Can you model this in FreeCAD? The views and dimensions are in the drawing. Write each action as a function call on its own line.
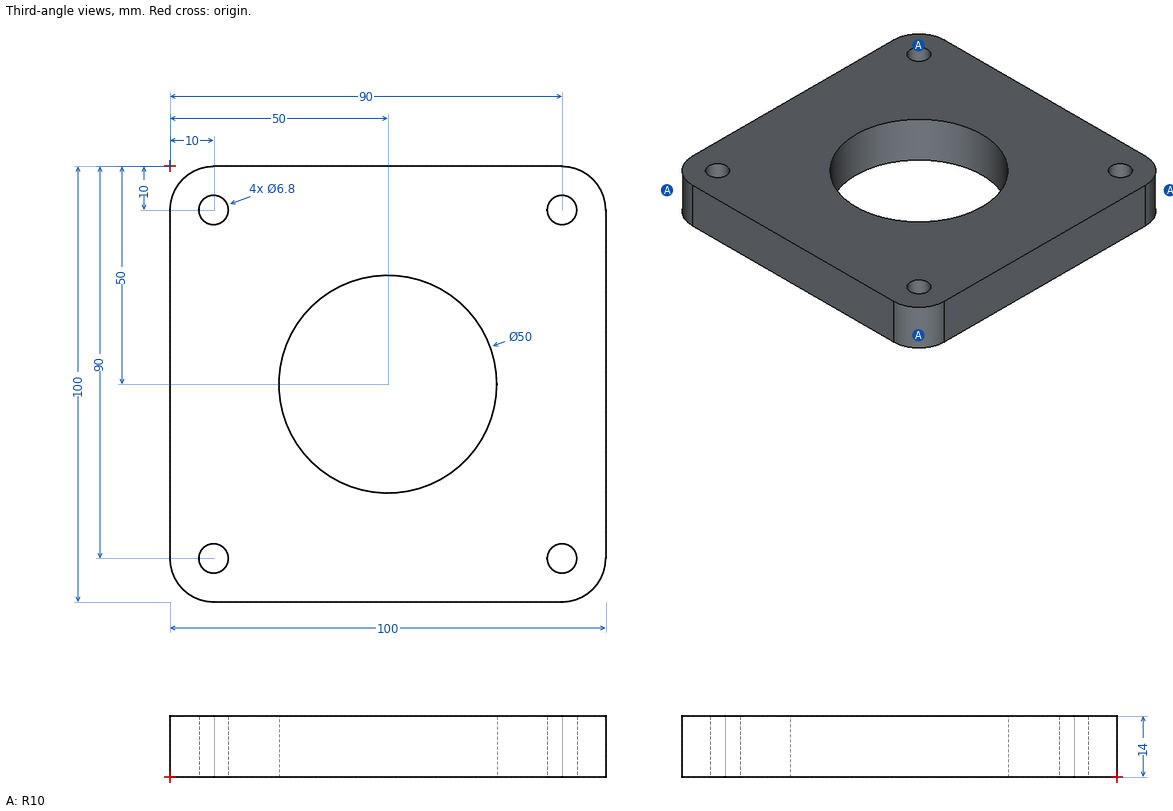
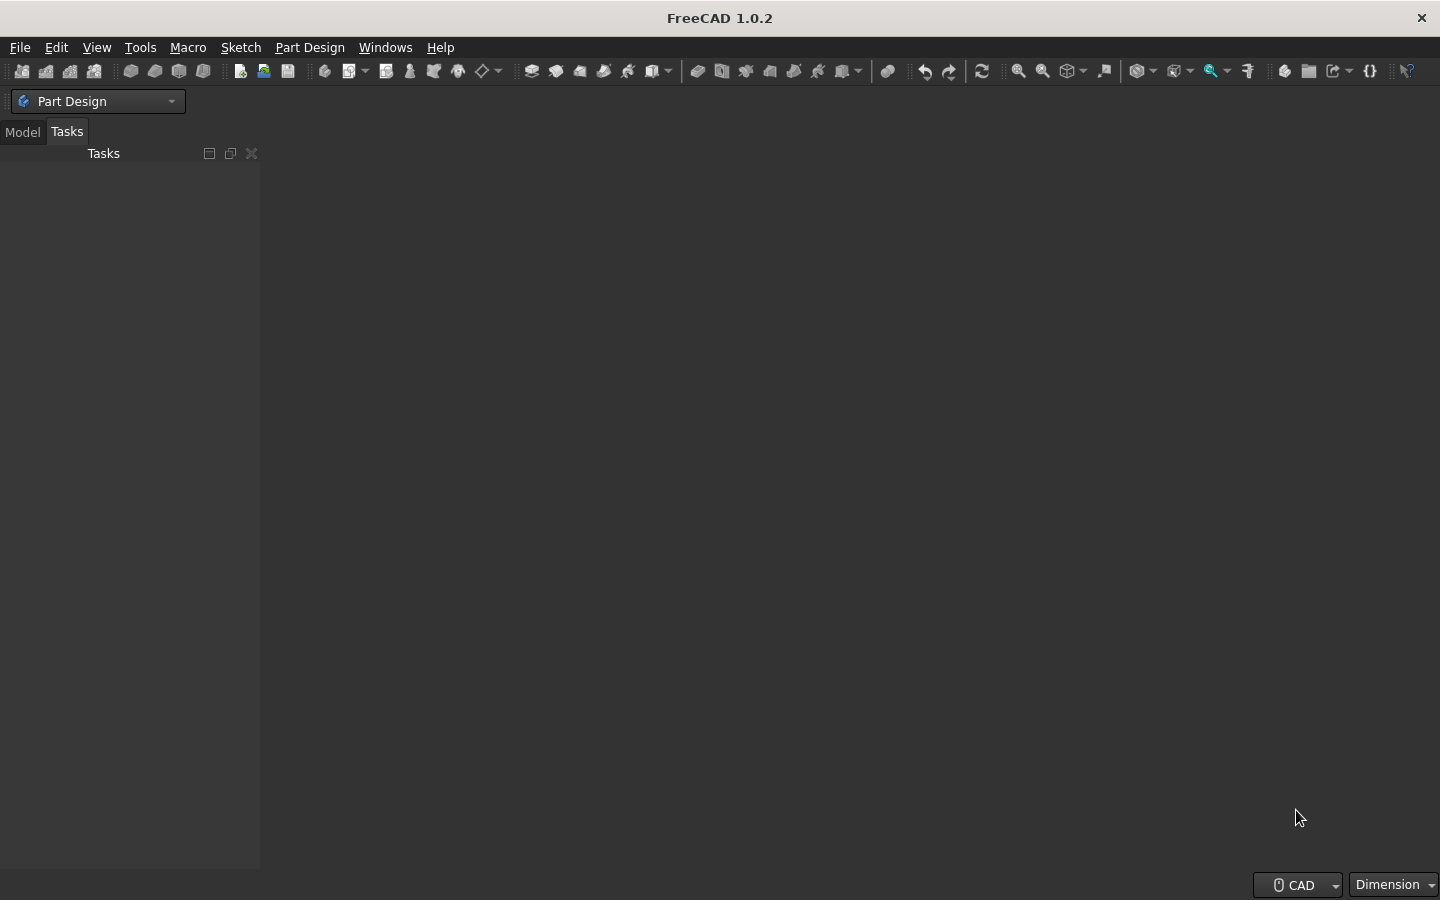
click(240, 72)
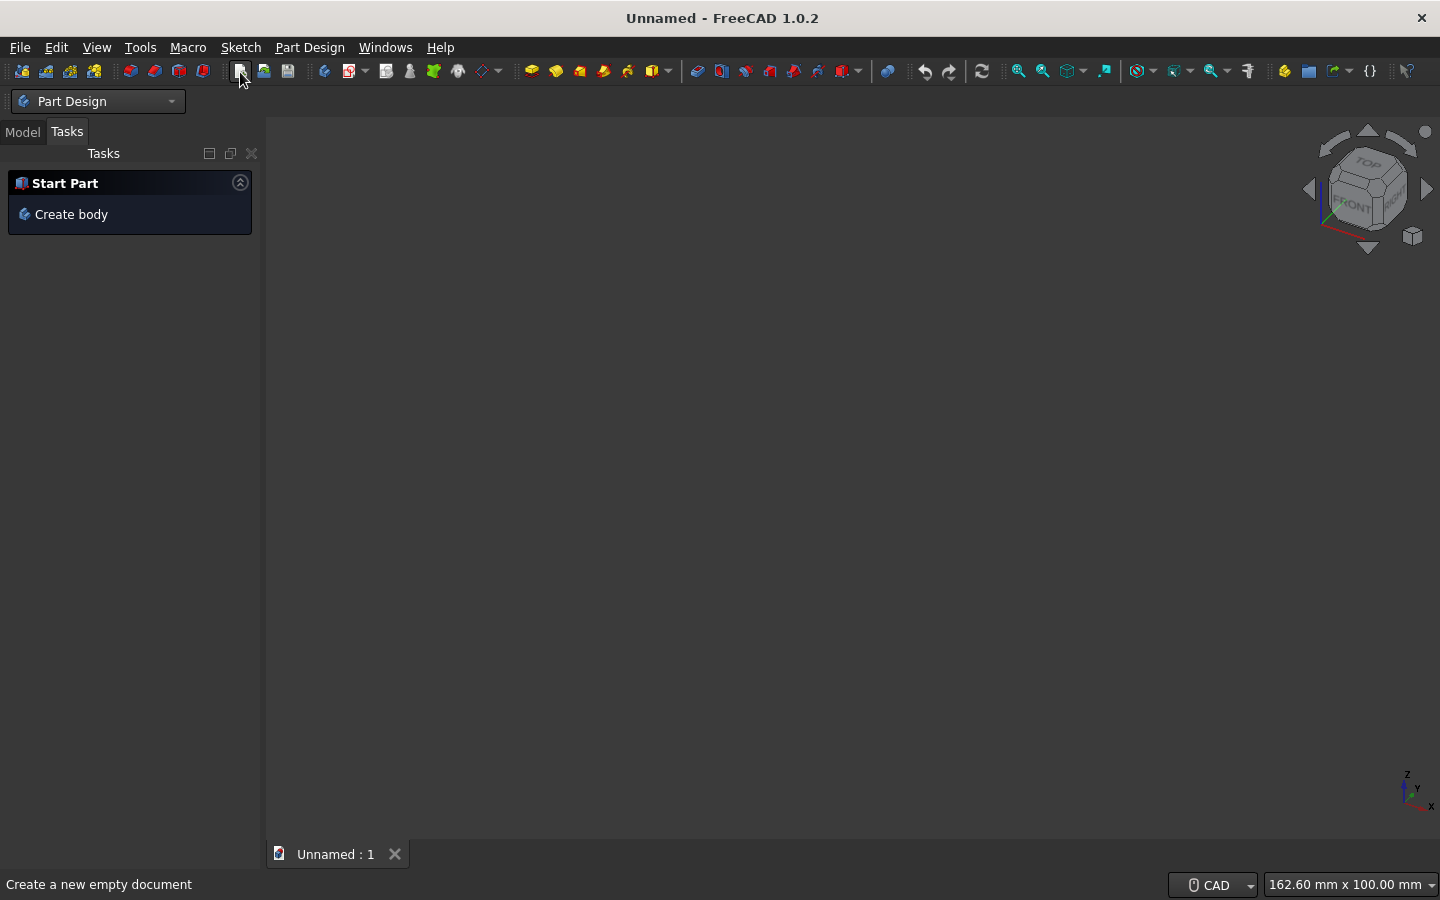
click(350, 72)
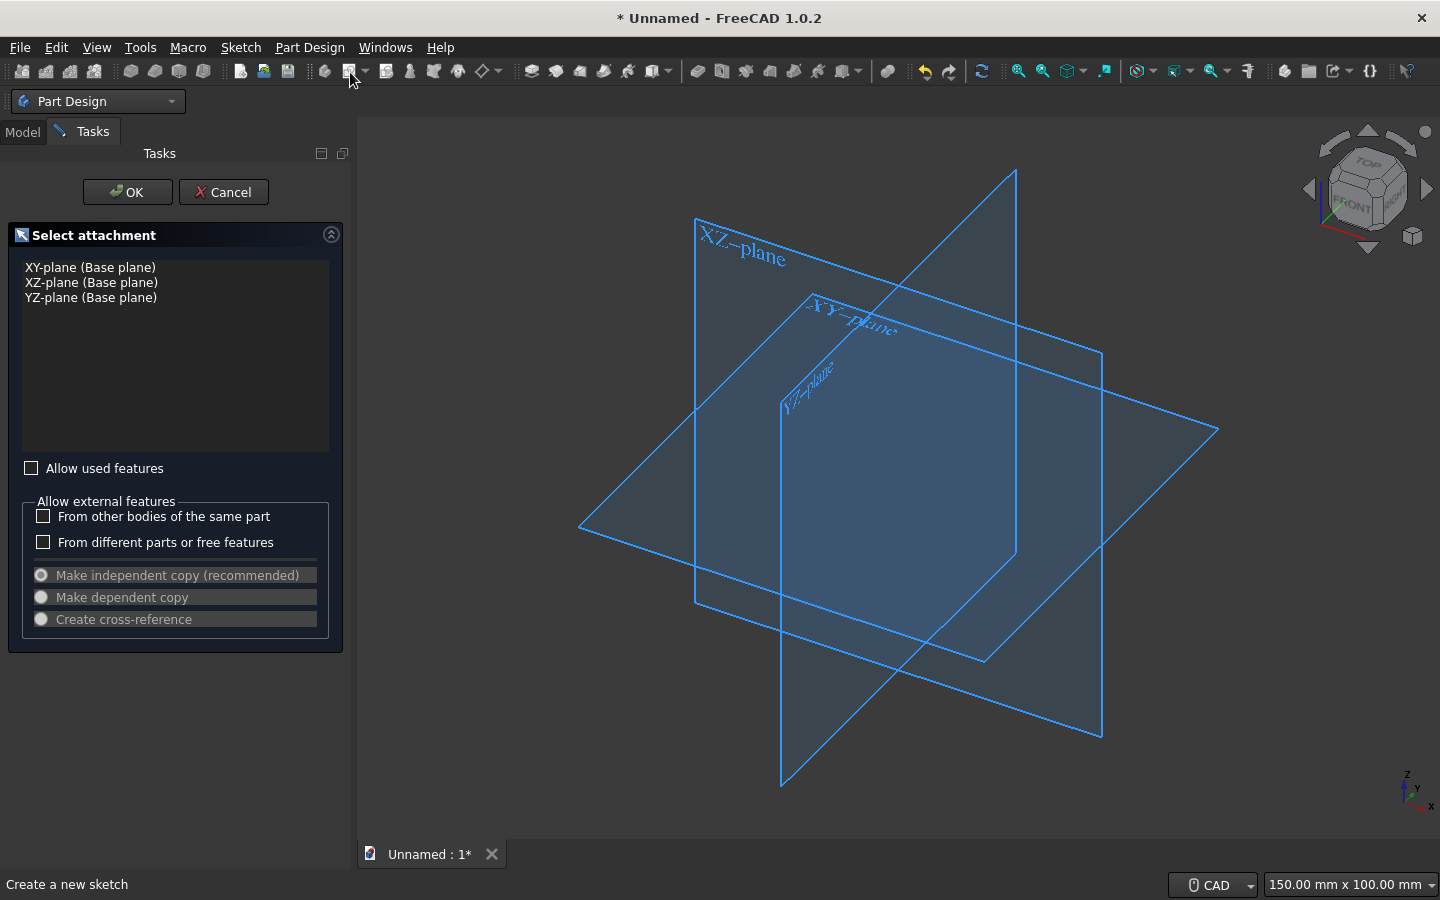
click(82, 268)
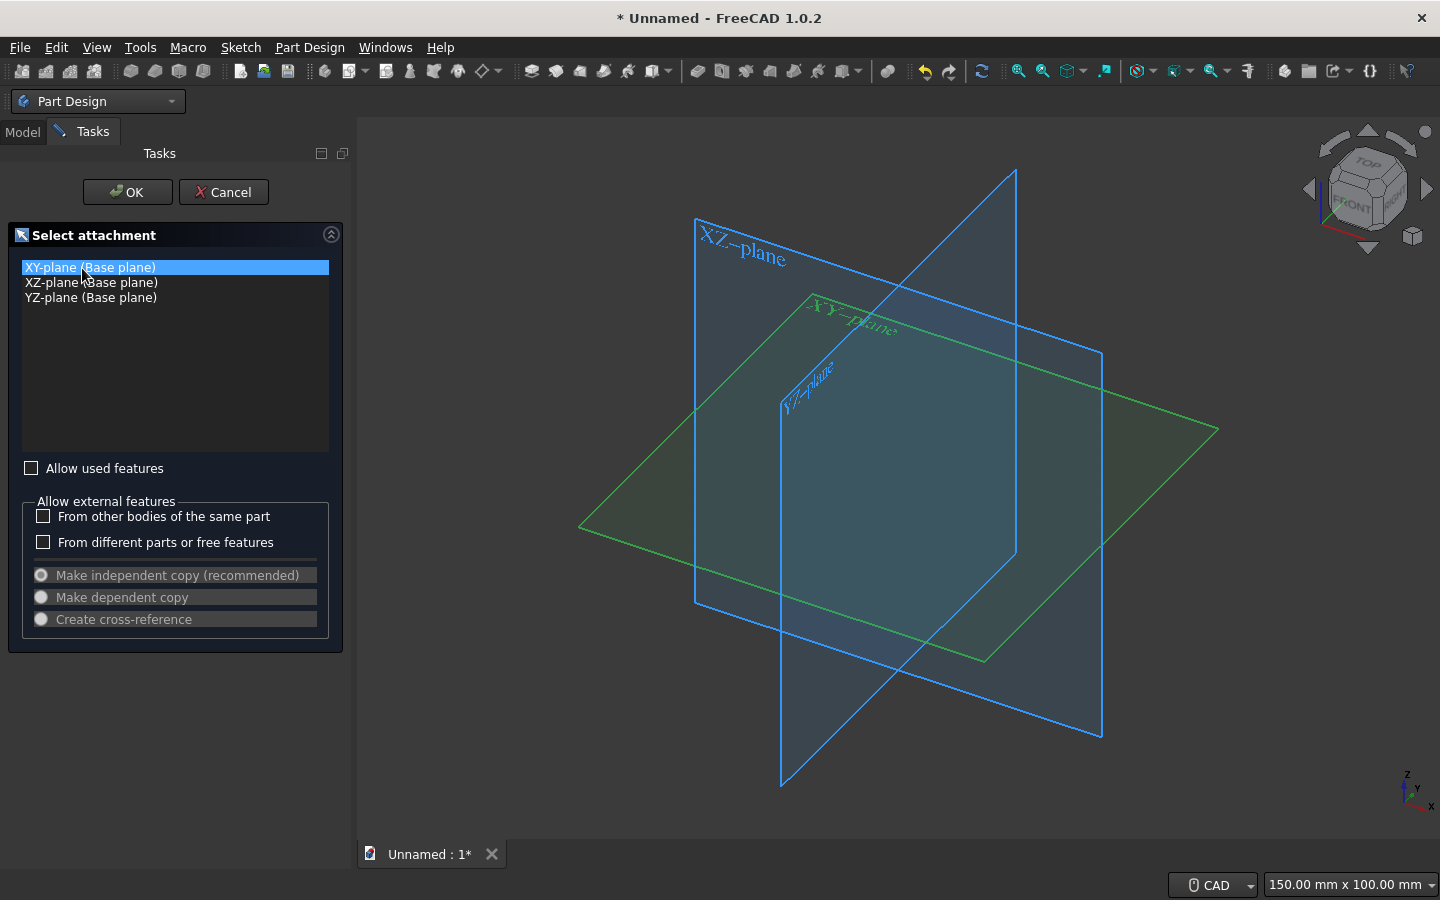
click(128, 192)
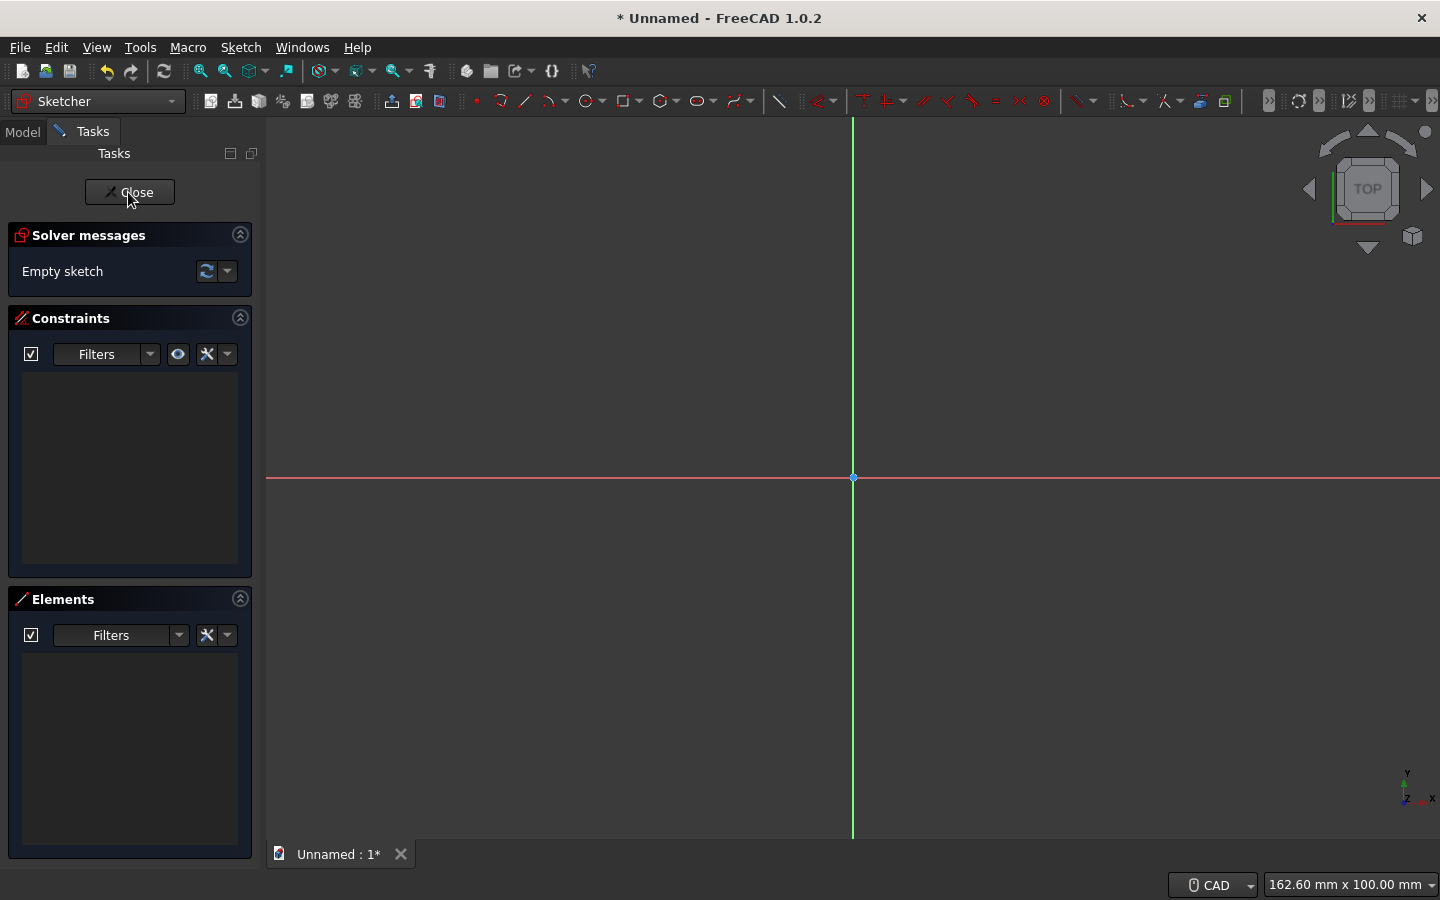
scroll(294, 145, down, 3)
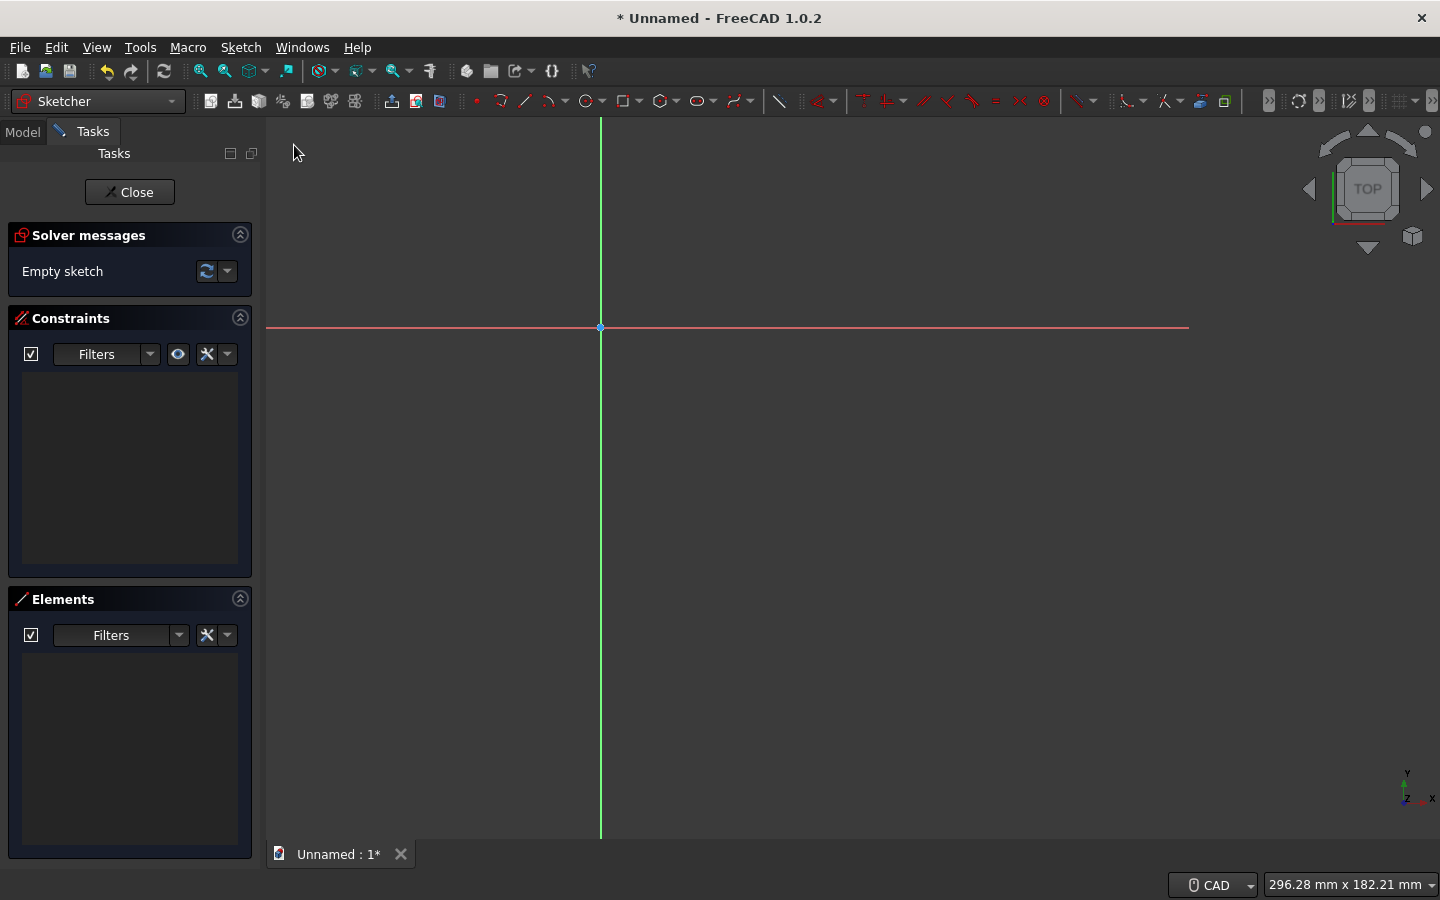
click(624, 102)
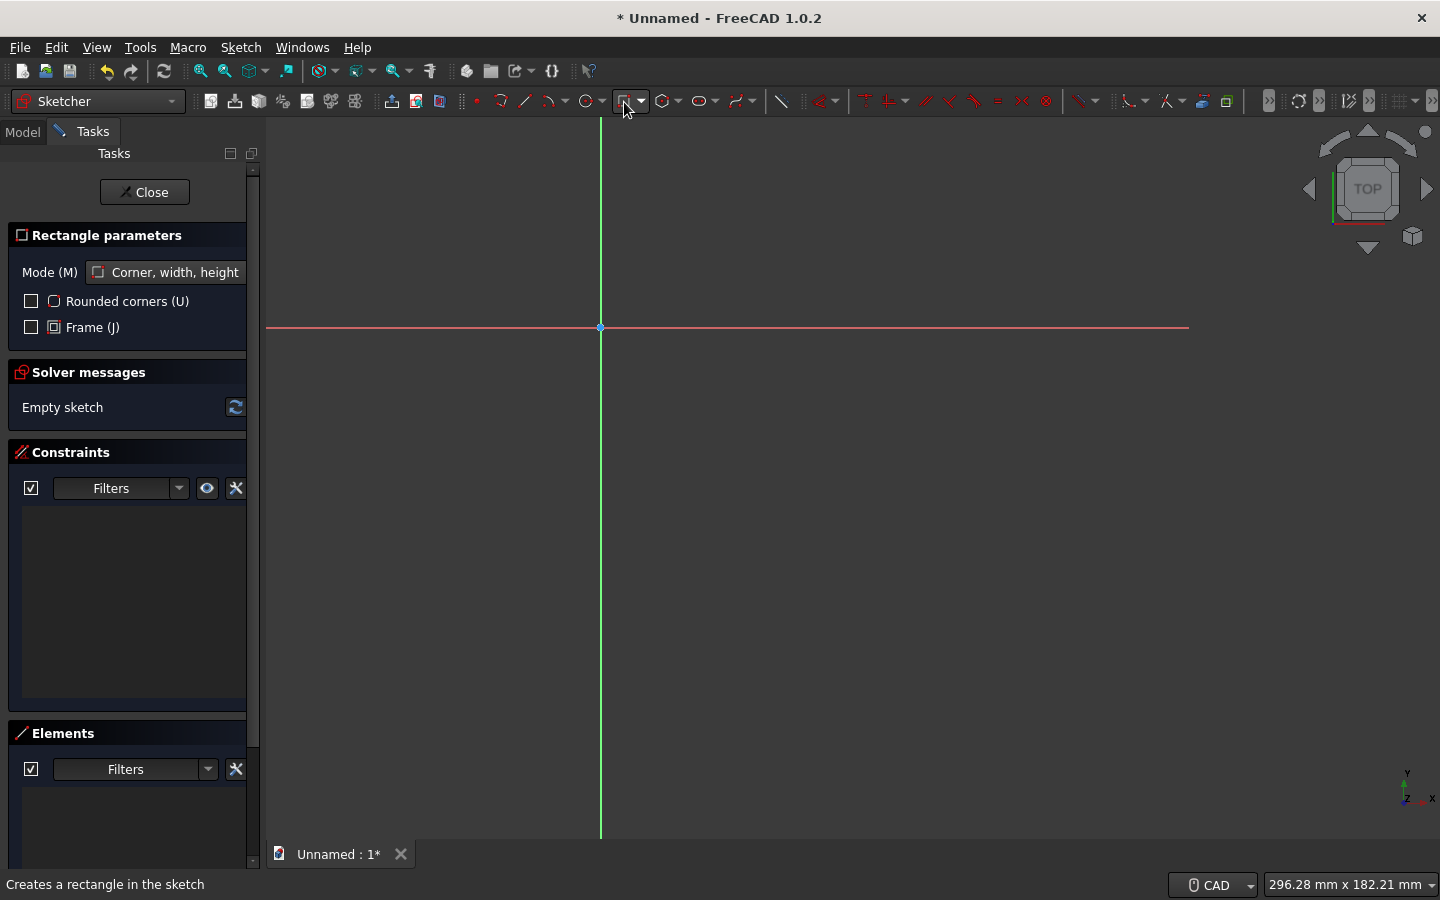
click(601, 328)
click(997, 724)
key(Escape)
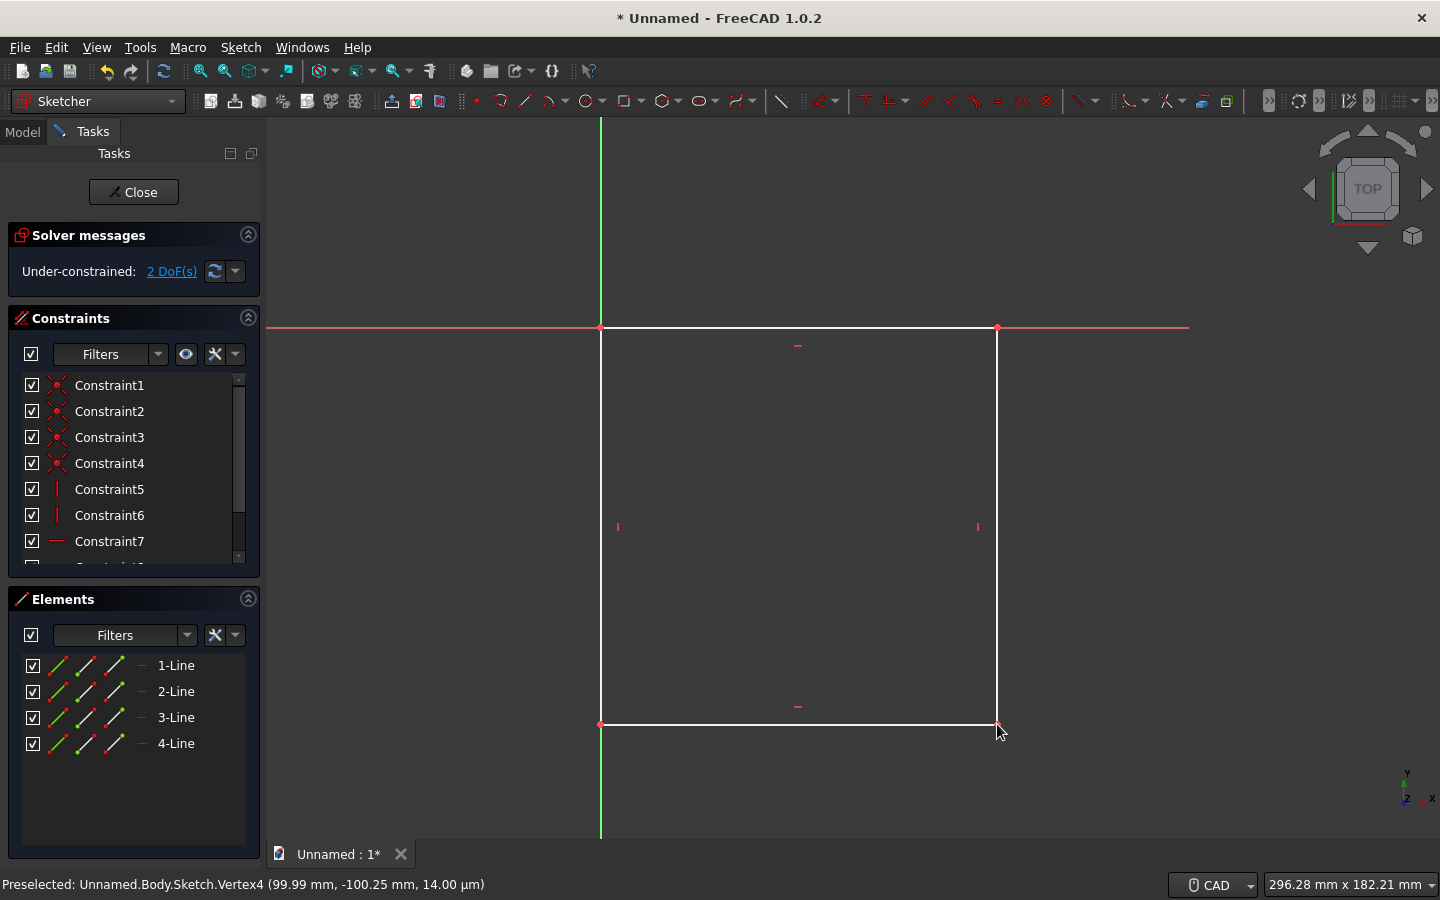
click(820, 102)